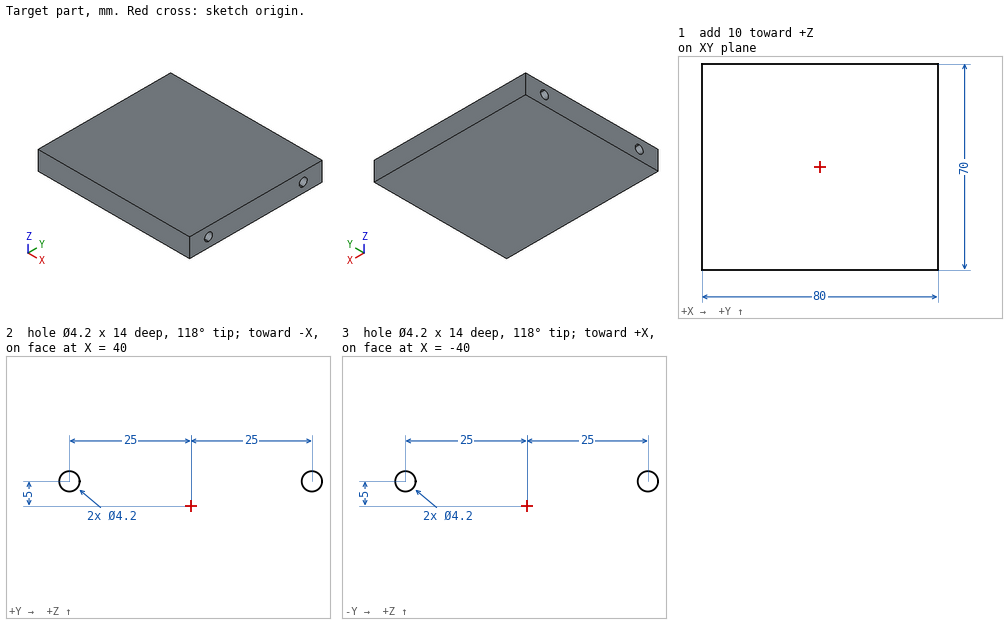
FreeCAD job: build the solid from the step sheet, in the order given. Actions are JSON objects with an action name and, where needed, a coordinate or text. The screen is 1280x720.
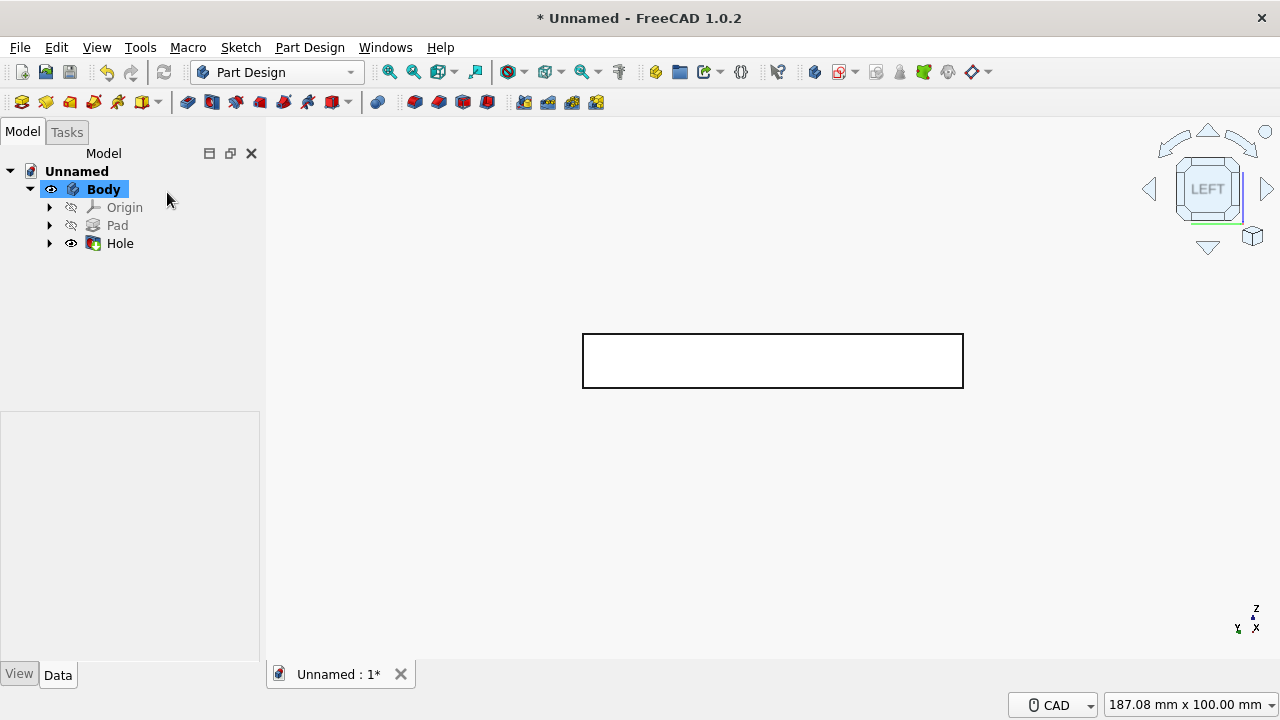
{"action": "left_click", "coordinate": [390, 72]}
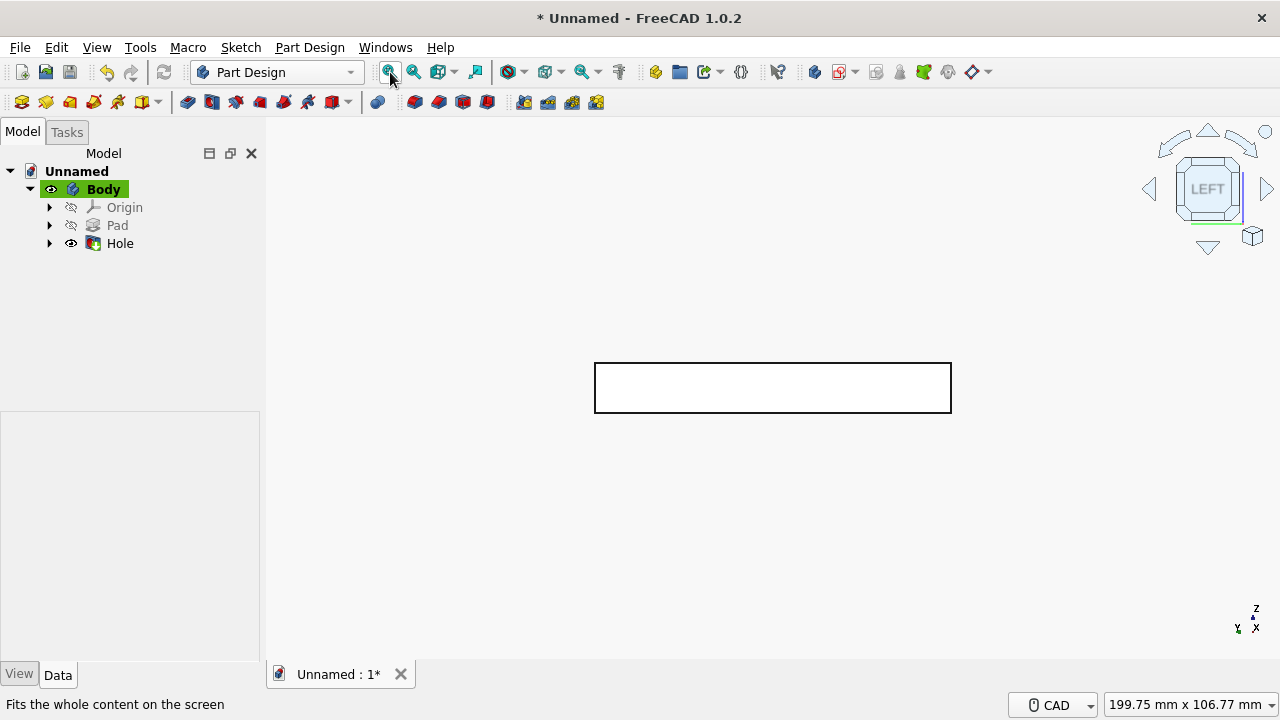
{"action": "left_click", "coordinate": [621, 387]}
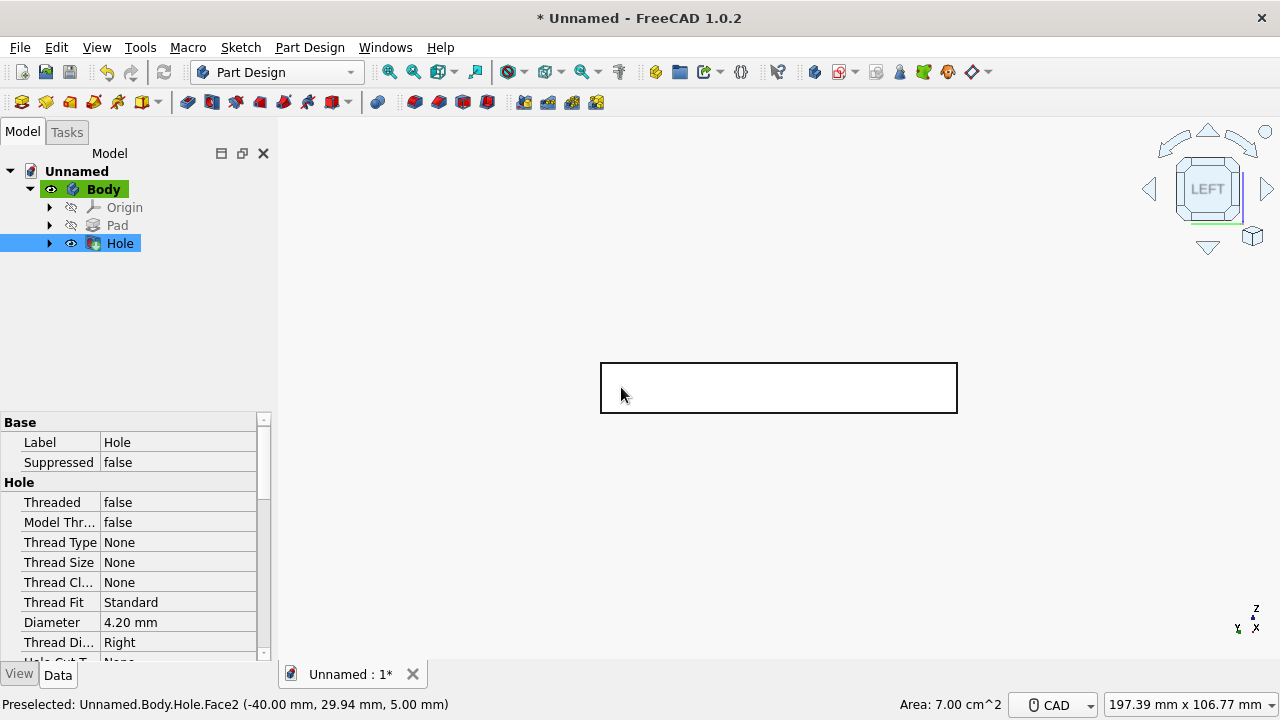
{"action": "left_click", "coordinate": [840, 72]}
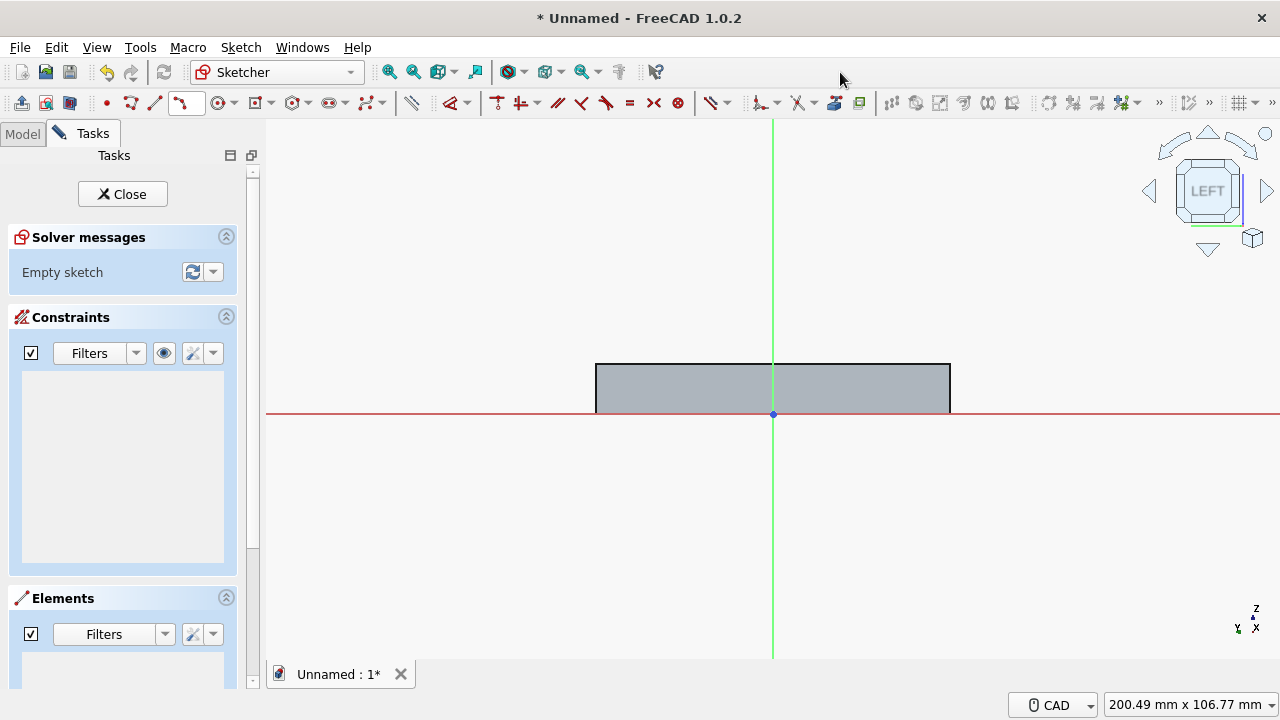
{"action": "scroll", "coordinate": [829, 402], "scroll_direction": "up", "scroll_amount": 4}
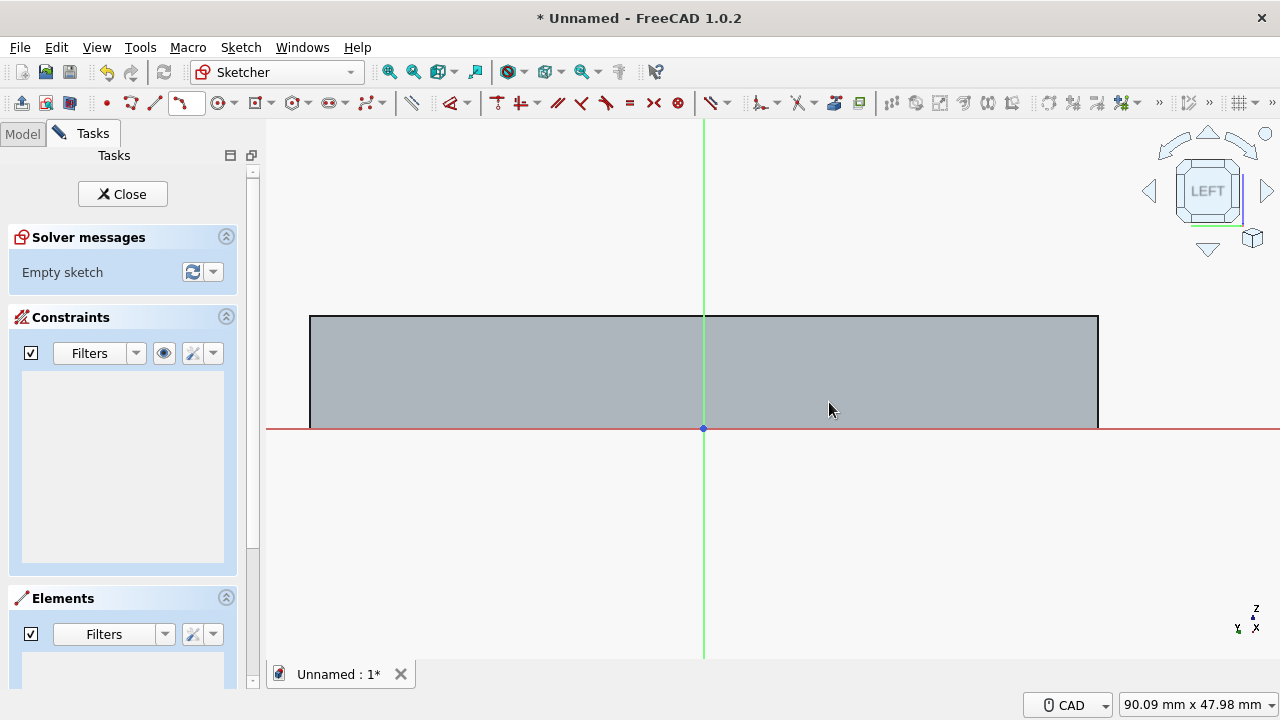
{"action": "key", "text": "g c"}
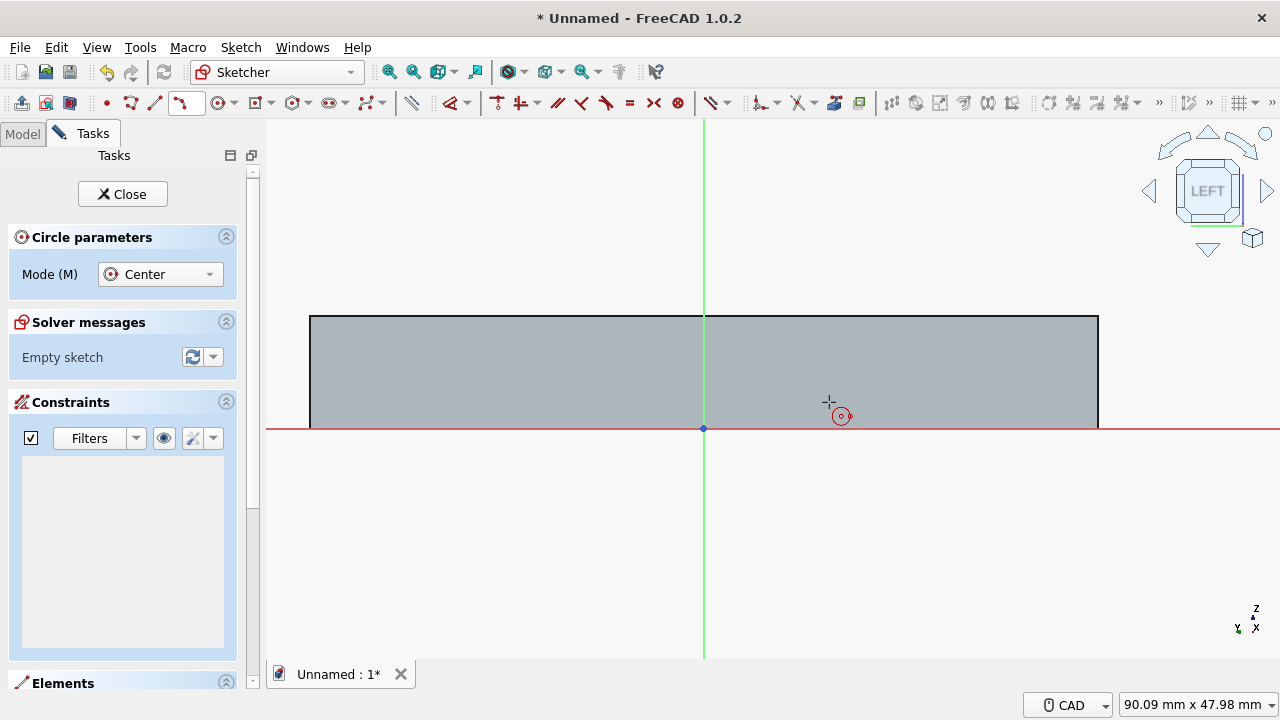
{"action": "left_click", "coordinate": [422, 372]}
{"action": "left_click", "coordinate": [439, 356]}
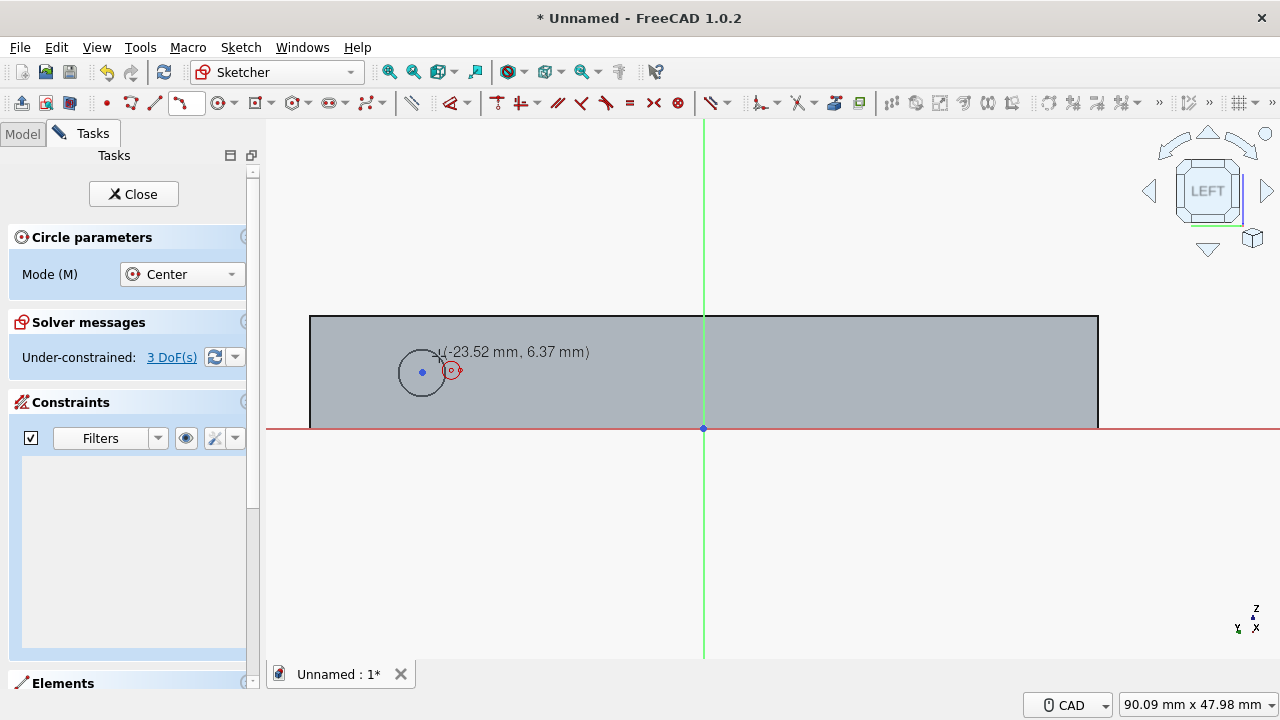
{"action": "left_click", "coordinate": [985, 372]}
{"action": "left_click", "coordinate": [1002, 356]}
{"action": "key", "text": "Escape"}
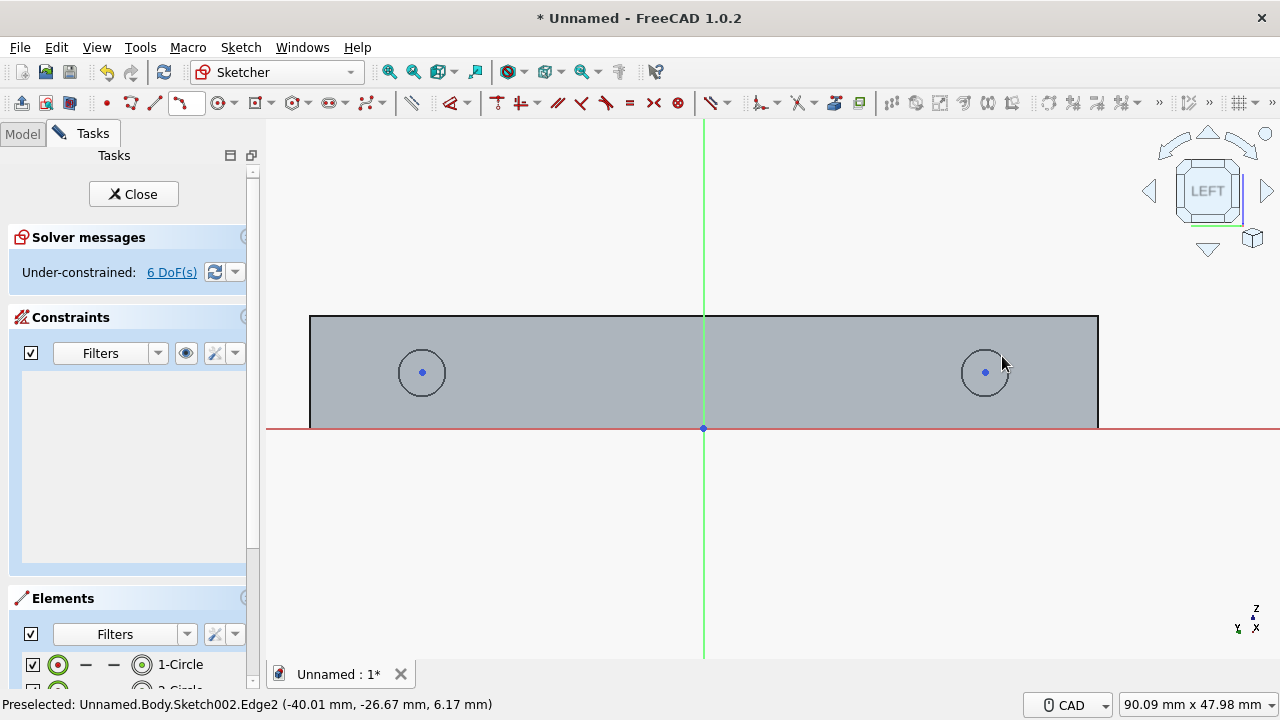
{"action": "left_click", "coordinate": [438, 356]}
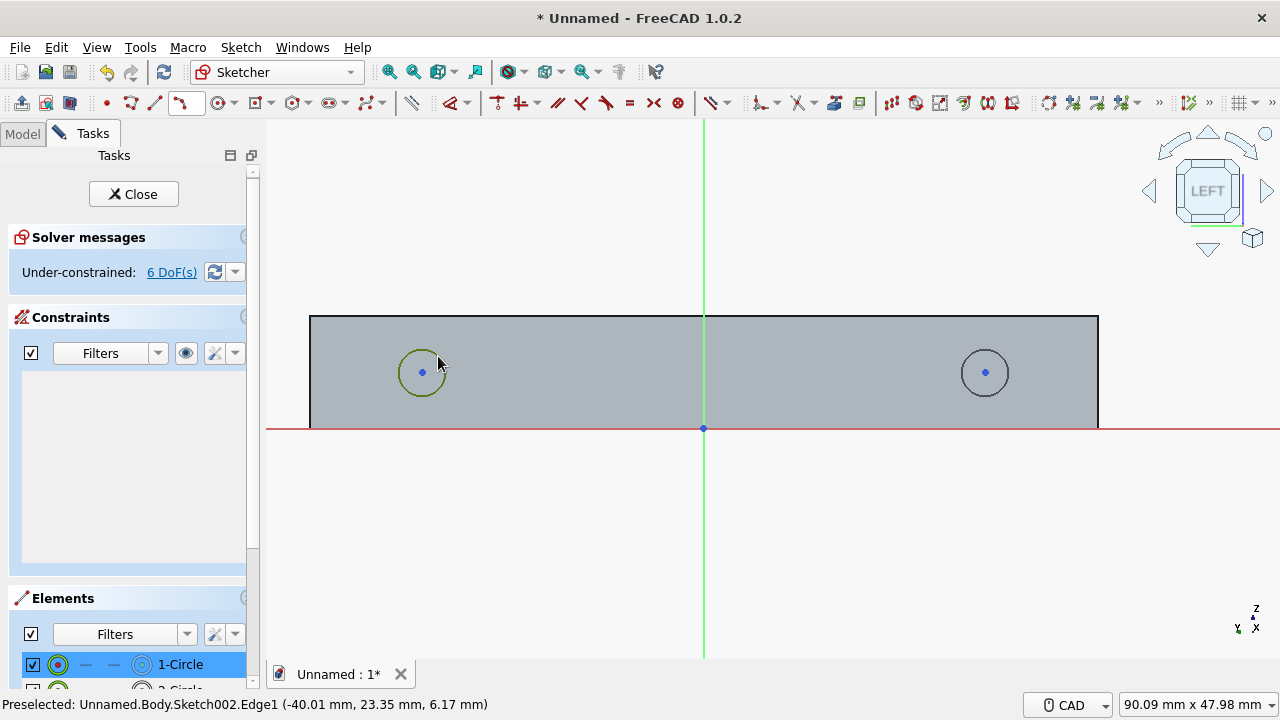
{"action": "left_click", "coordinate": [1001, 356]}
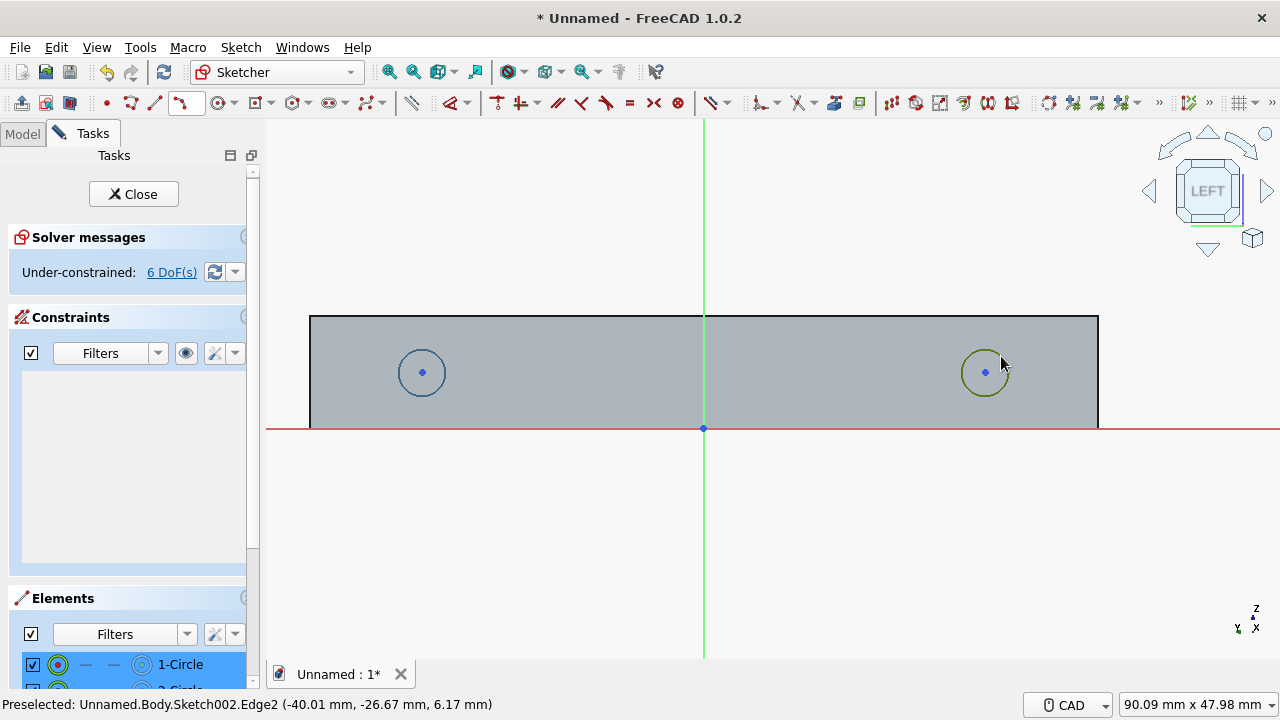
{"action": "key", "text": "e"}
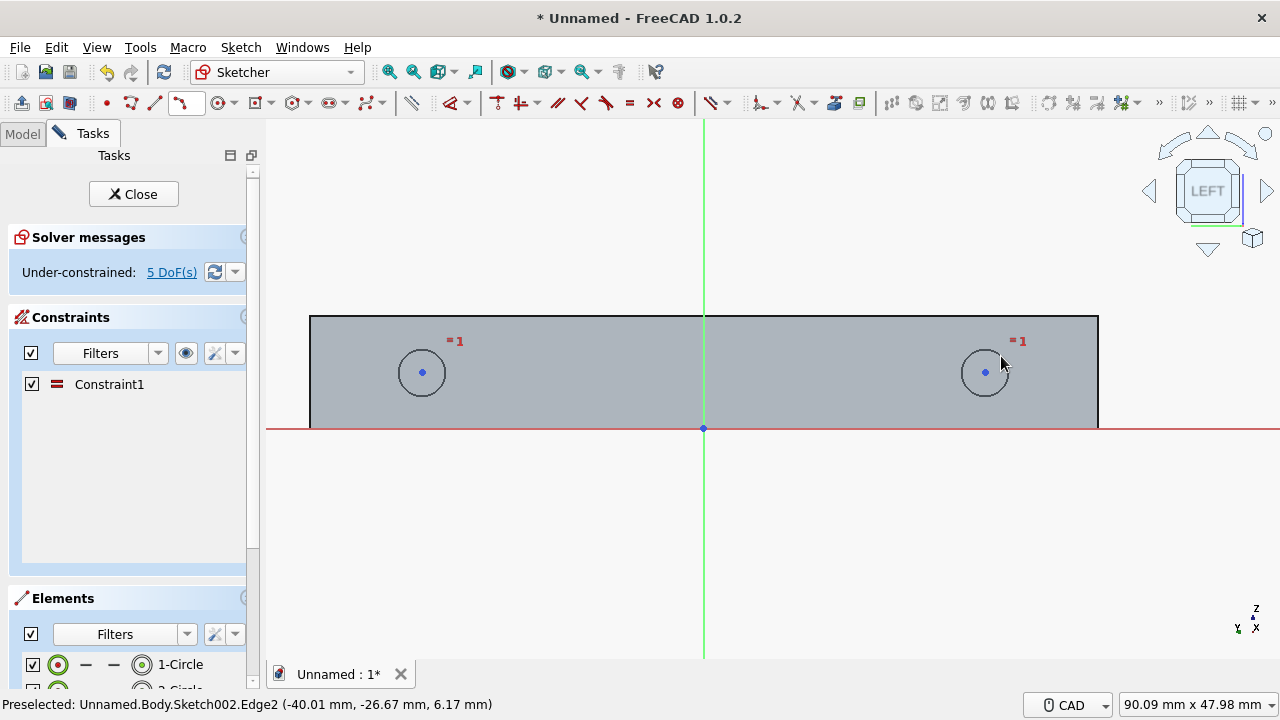
{"action": "left_click", "coordinate": [422, 373]}